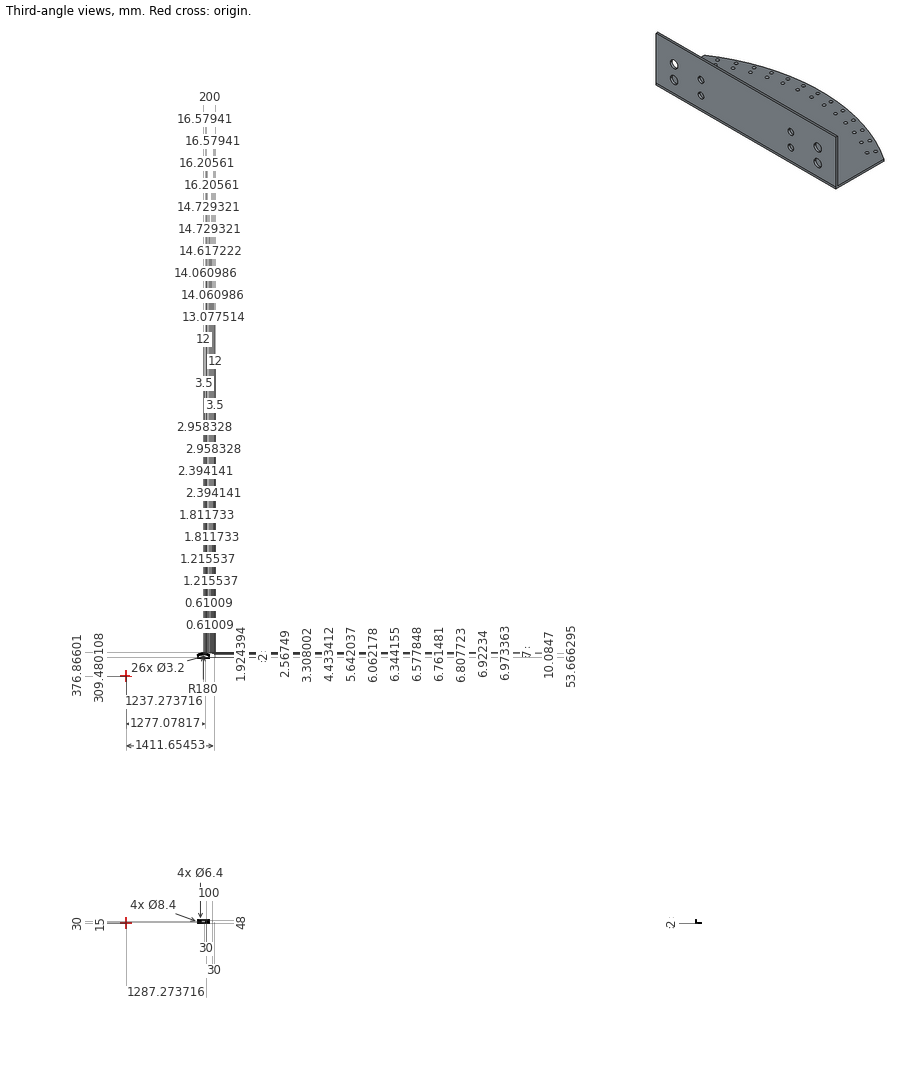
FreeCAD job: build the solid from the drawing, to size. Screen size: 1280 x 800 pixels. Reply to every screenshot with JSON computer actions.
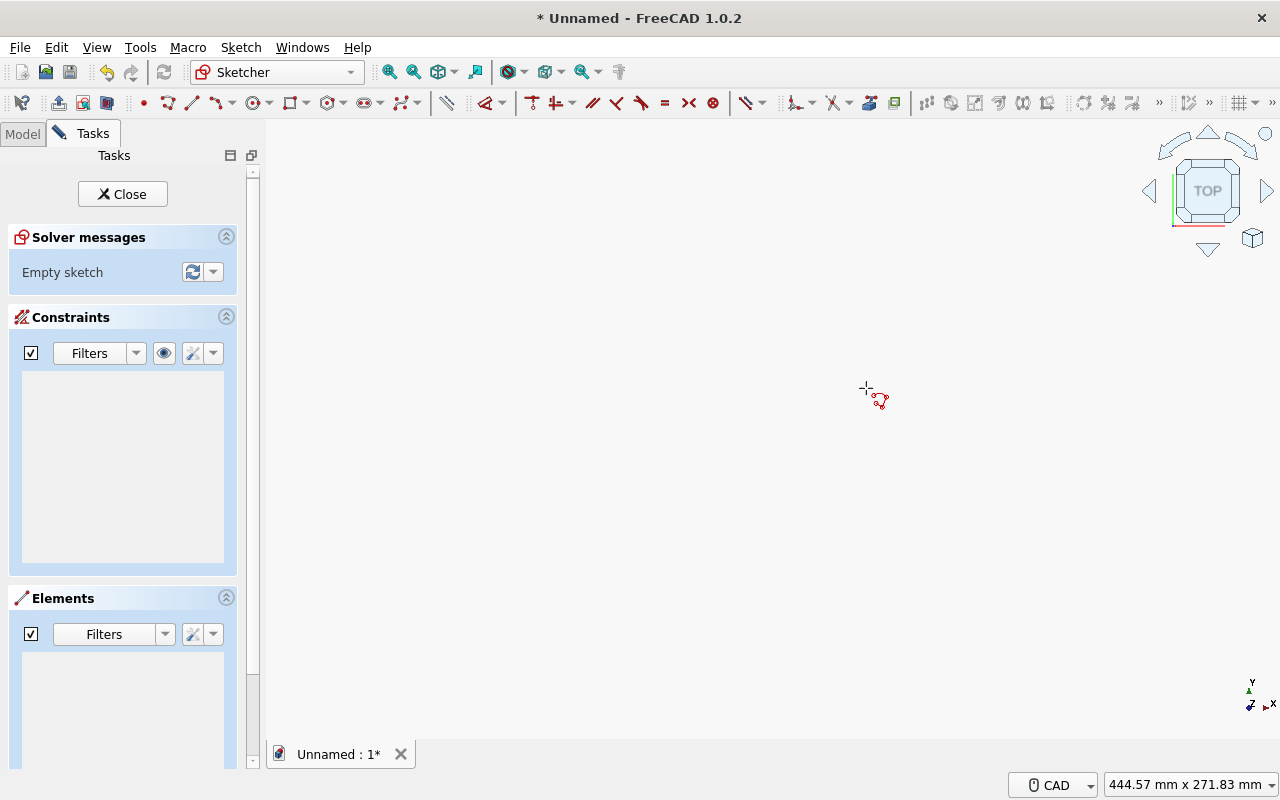
{"action": "left_click", "coordinate": [457, 389]}
{"action": "left_click", "coordinate": [457, 512]}
{"action": "left_click", "coordinate": [913, 512]}
{"action": "left_click", "coordinate": [913, 389]}
{"action": "right_click", "coordinate": [913, 389]}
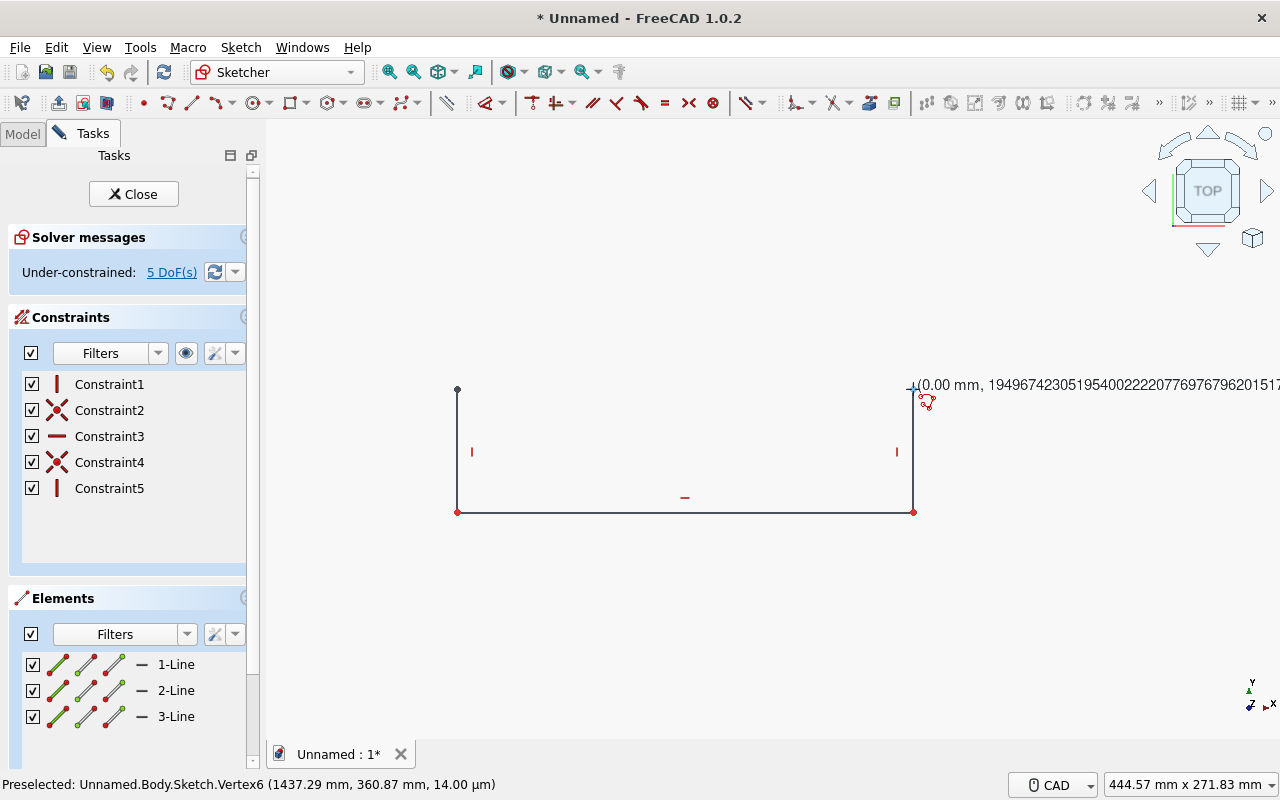
{"action": "key", "text": "g 3 a"}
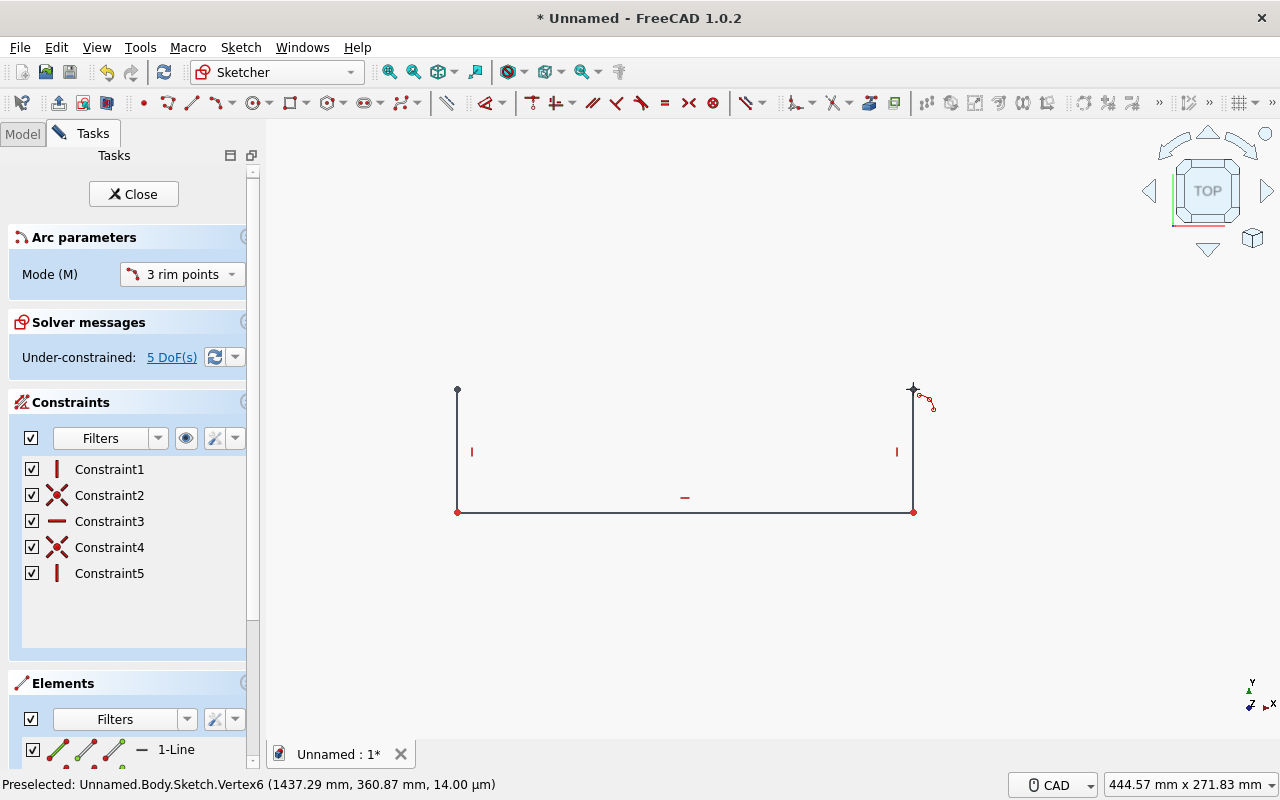
{"action": "left_click", "coordinate": [913, 390]}
{"action": "left_click", "coordinate": [457, 390]}
{"action": "left_click", "coordinate": [685, 320]}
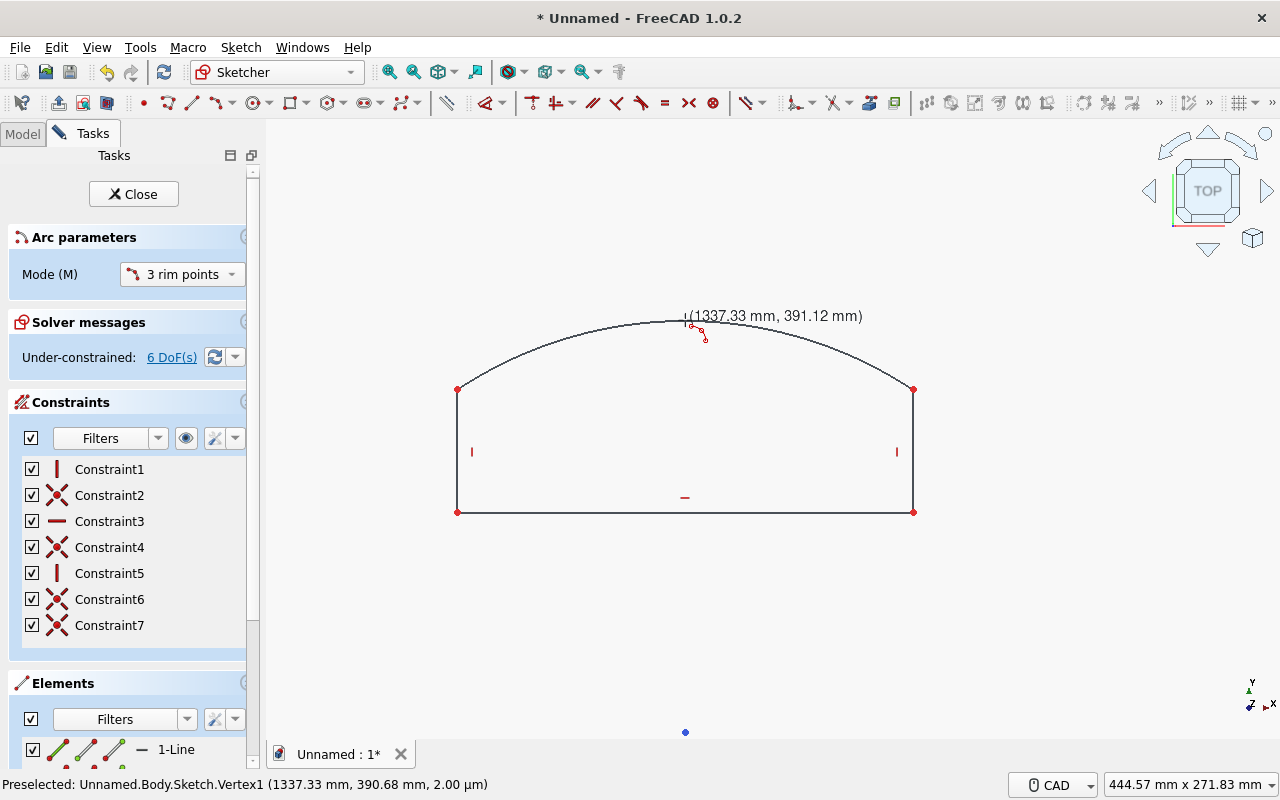
{"action": "left_click", "coordinate": [254, 104]}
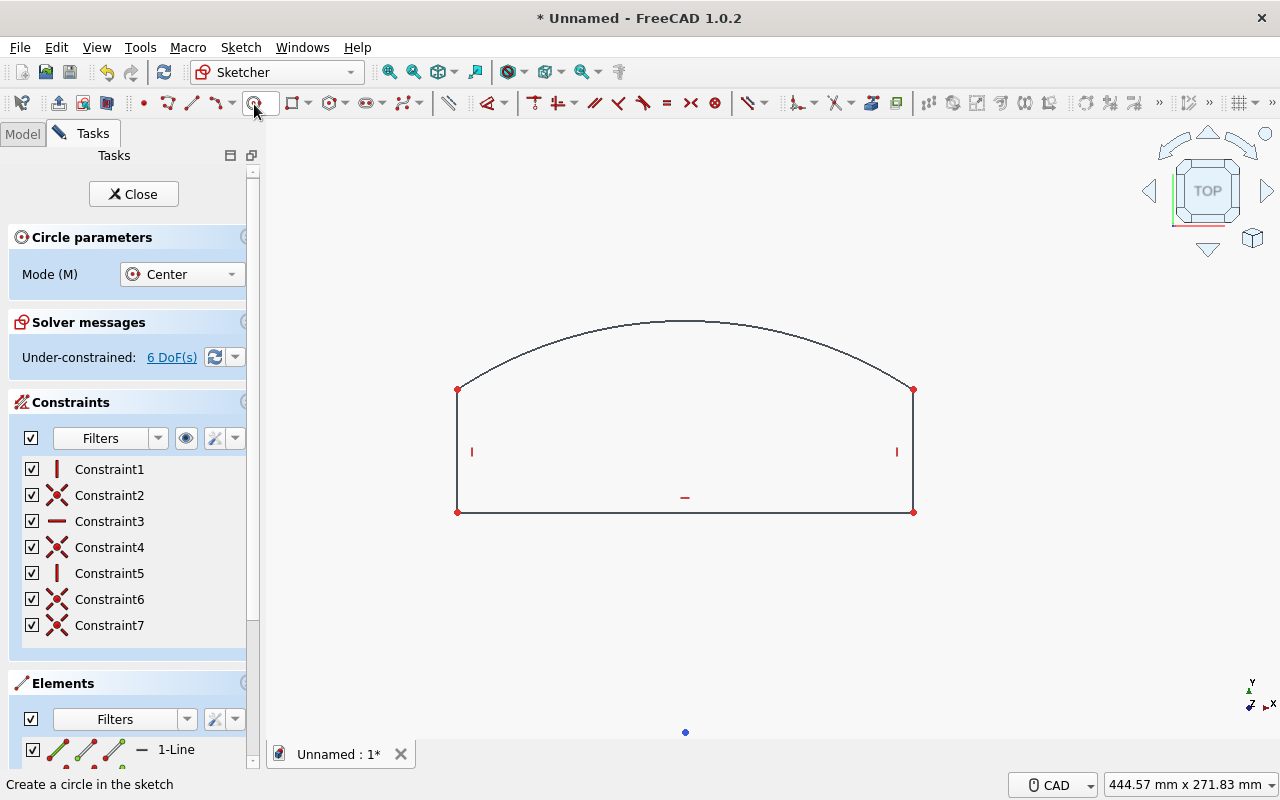
{"action": "scroll", "coordinate": [878, 397], "scroll_direction": "up", "scroll_amount": 10}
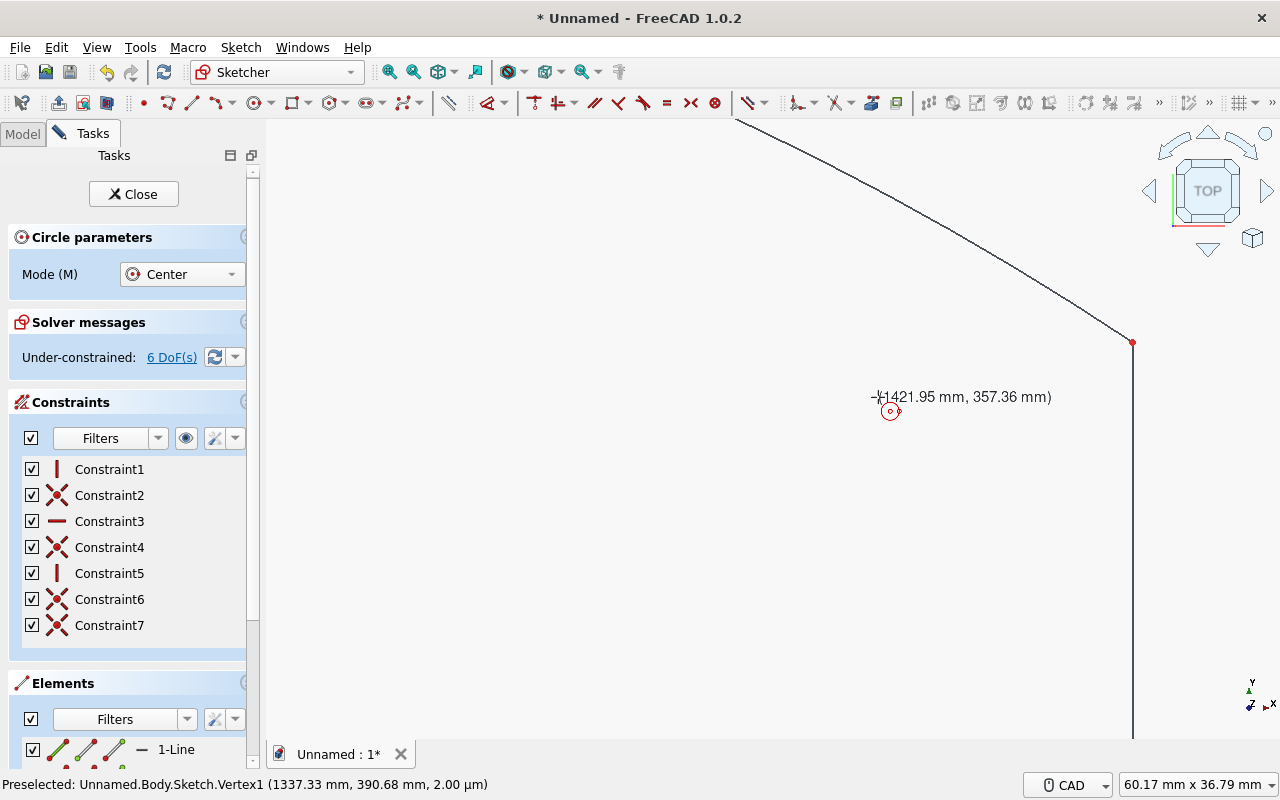
{"action": "scroll", "coordinate": [954, 408], "scroll_direction": "down", "scroll_amount": 9}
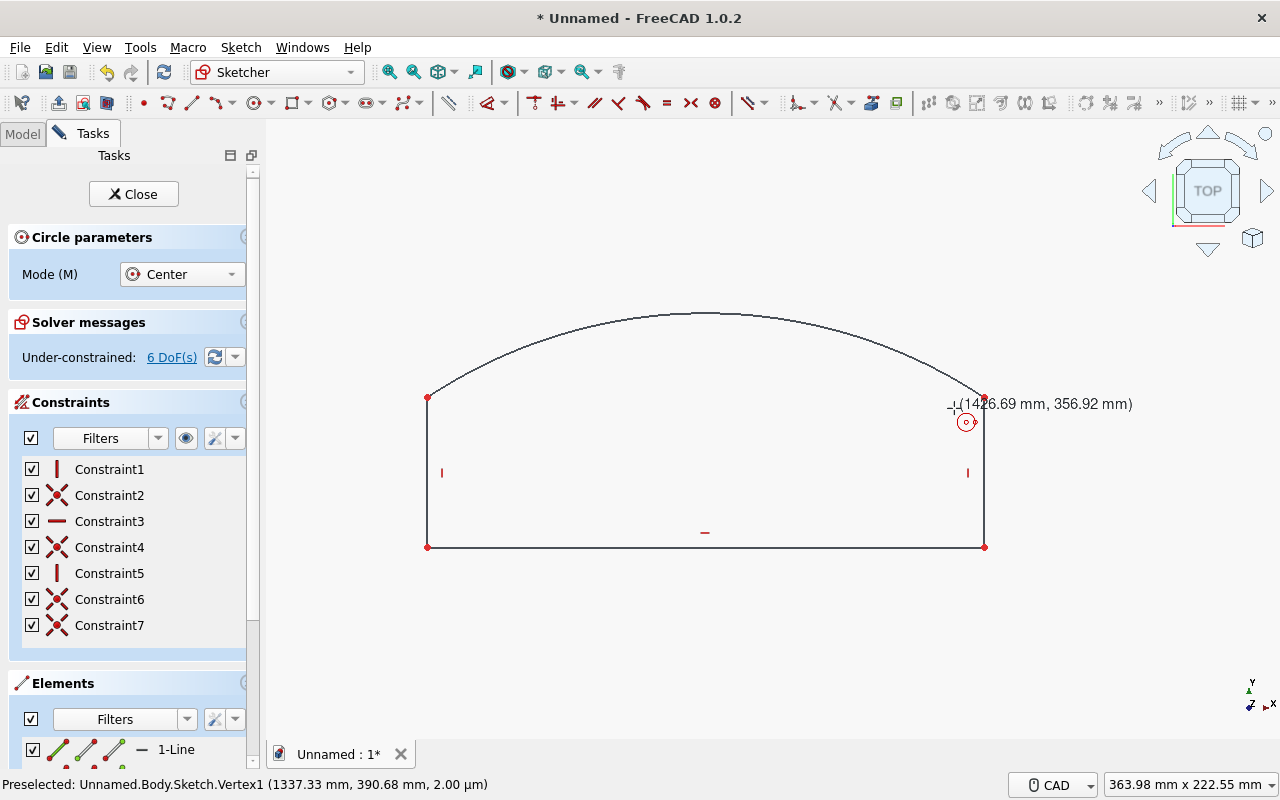
{"action": "left_click", "coordinate": [941, 406]}
{"action": "mouse_move", "coordinate": [944, 403]}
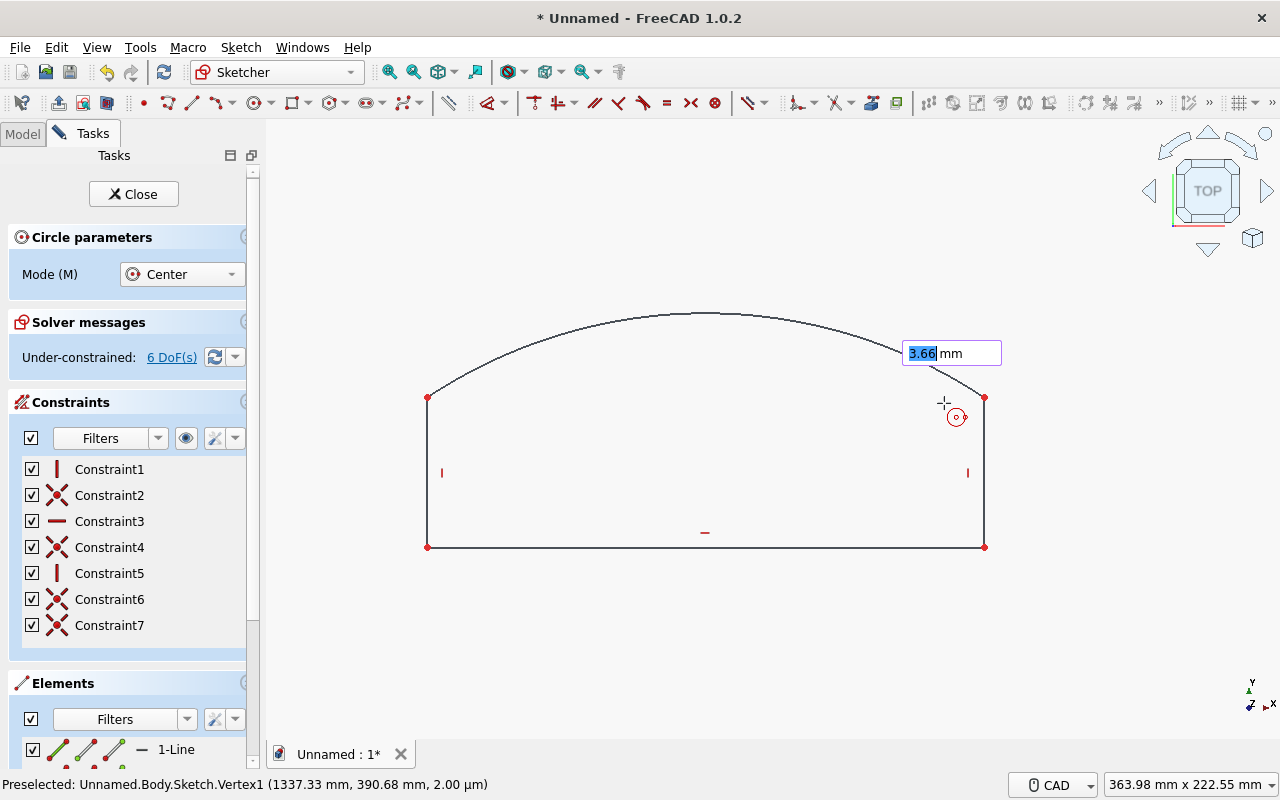
{"action": "type", "text": "3.2"}
{"action": "key", "text": "Return"}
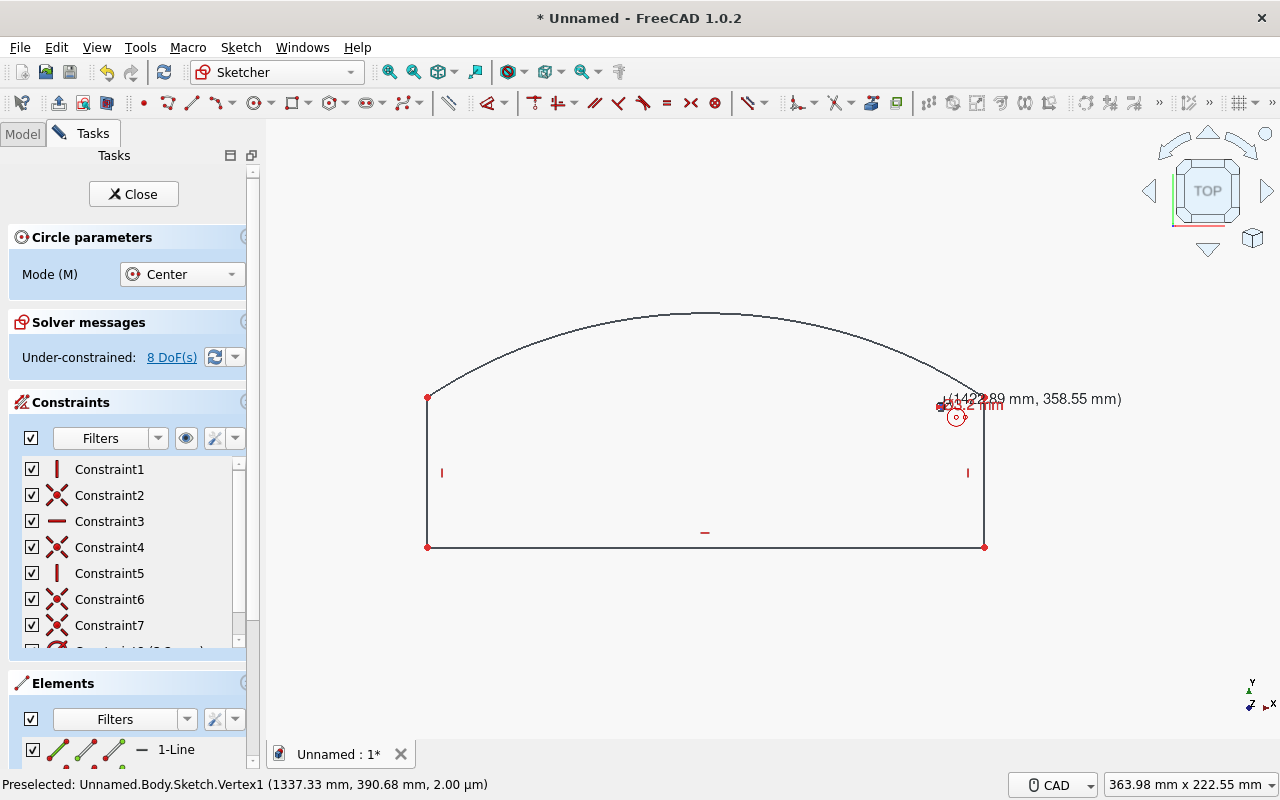
{"action": "scroll", "coordinate": [951, 389], "scroll_direction": "up", "scroll_amount": 9}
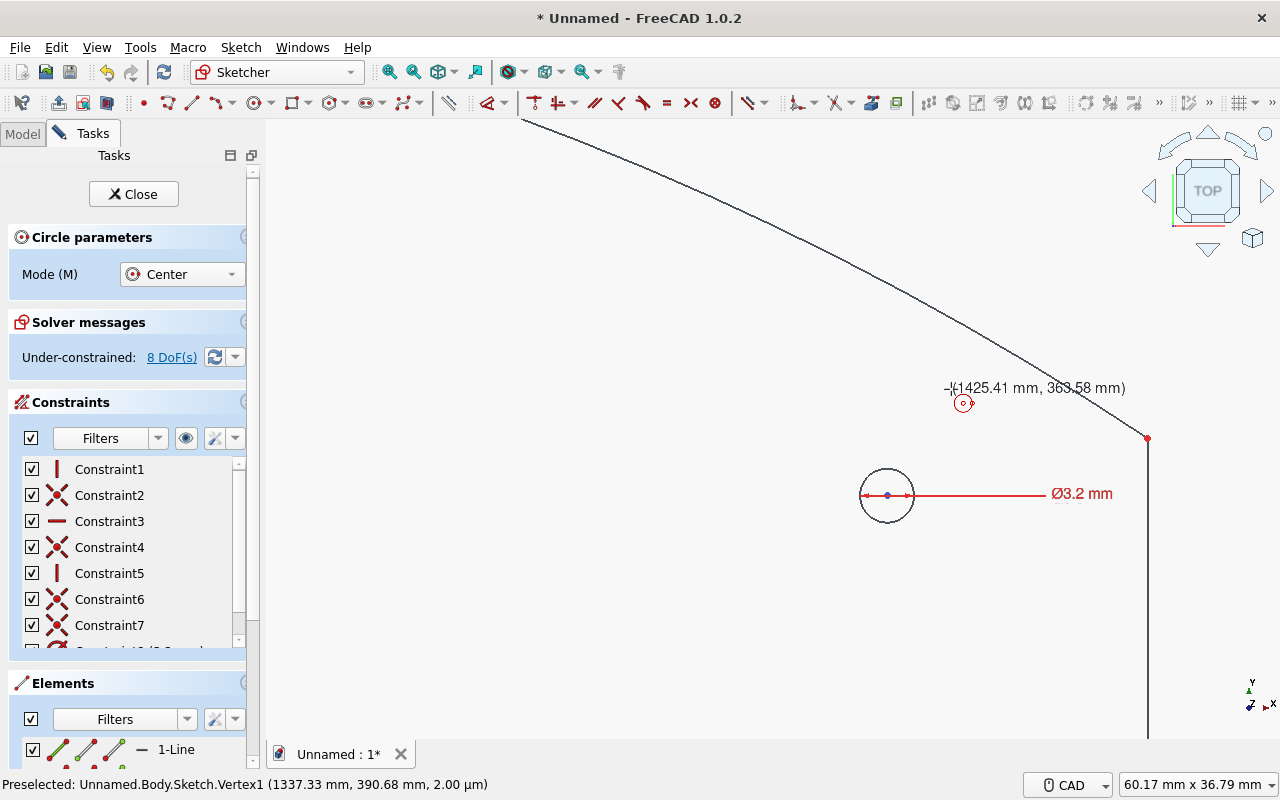
{"action": "scroll", "coordinate": [951, 389], "scroll_direction": "down", "scroll_amount": 9}